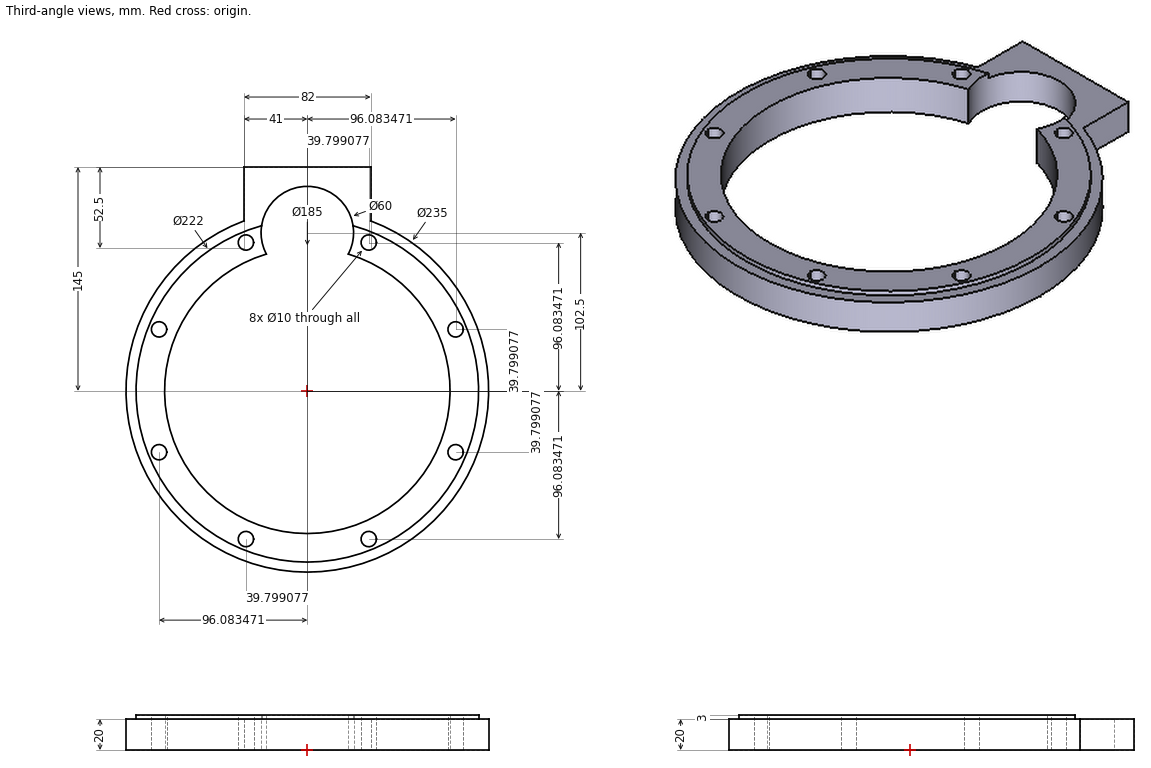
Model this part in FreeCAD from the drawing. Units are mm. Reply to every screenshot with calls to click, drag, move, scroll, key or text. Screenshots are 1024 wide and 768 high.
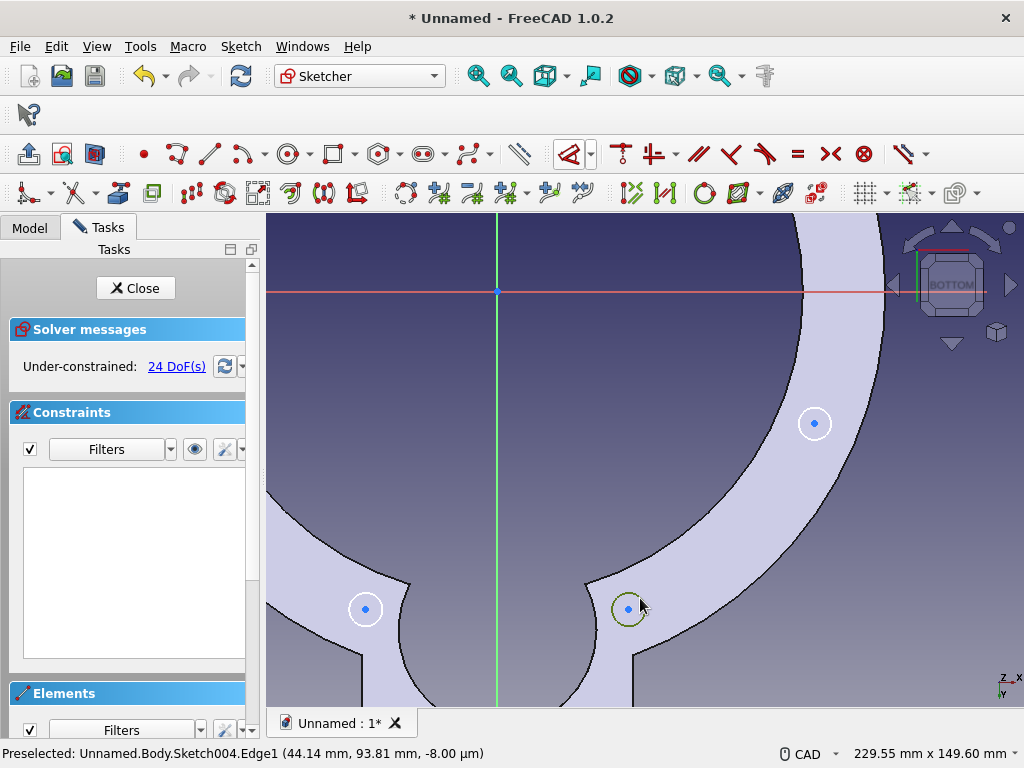
click(826, 412)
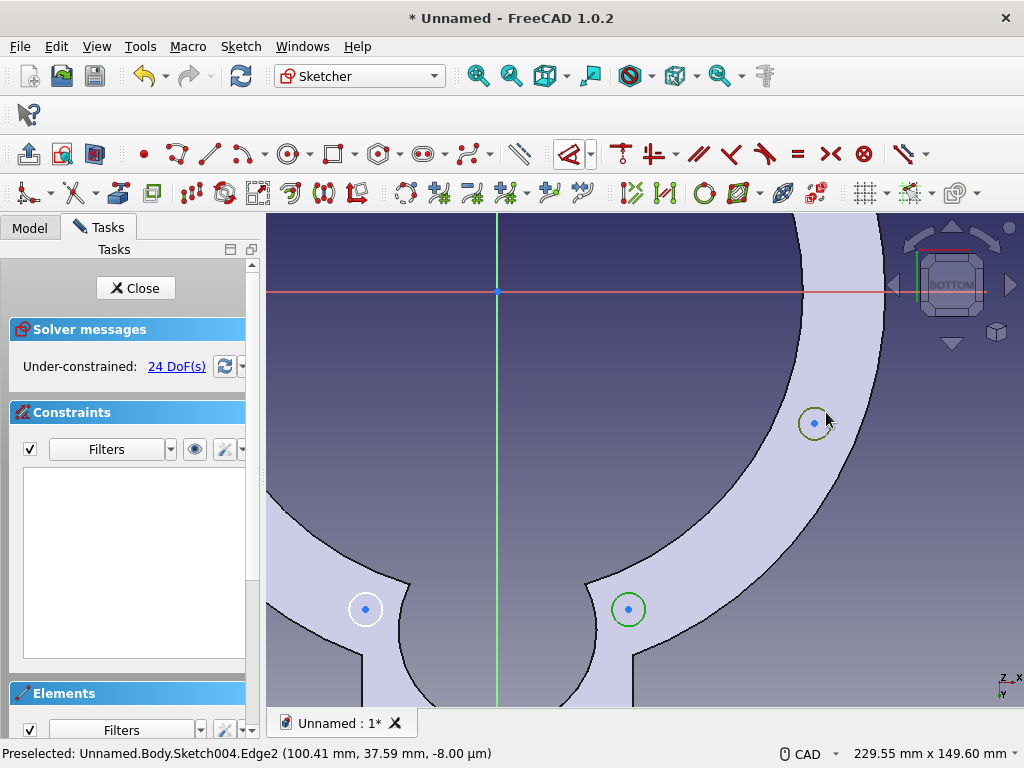
scroll(641, 597, down, 4)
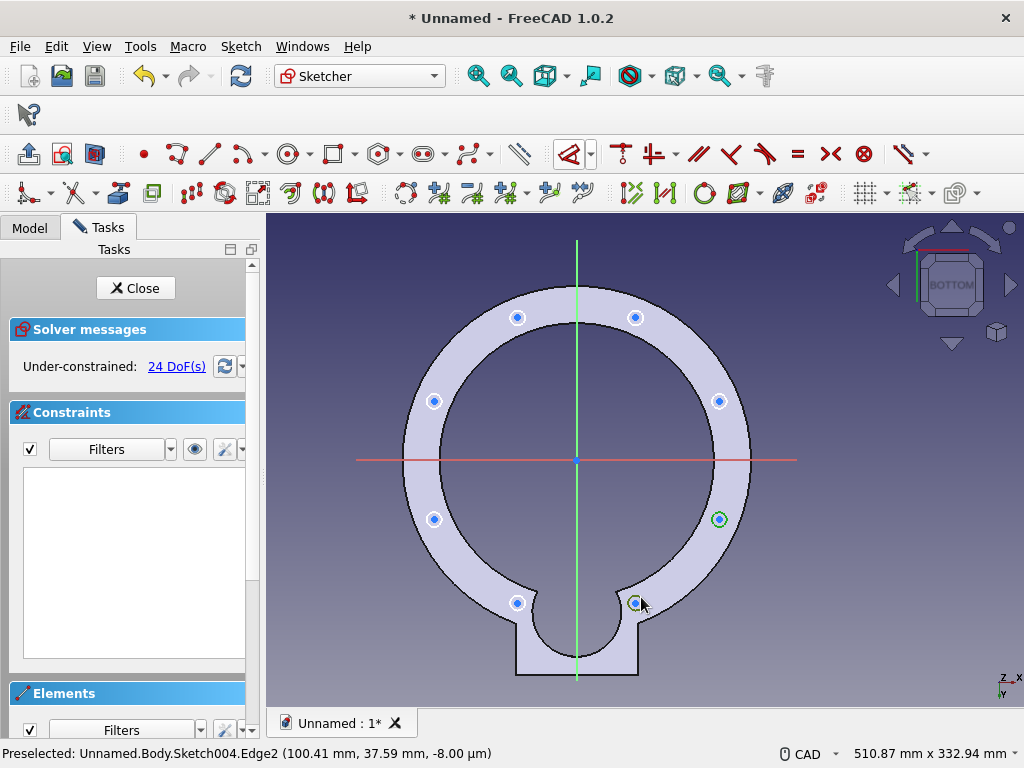
scroll(725, 396, up, 4)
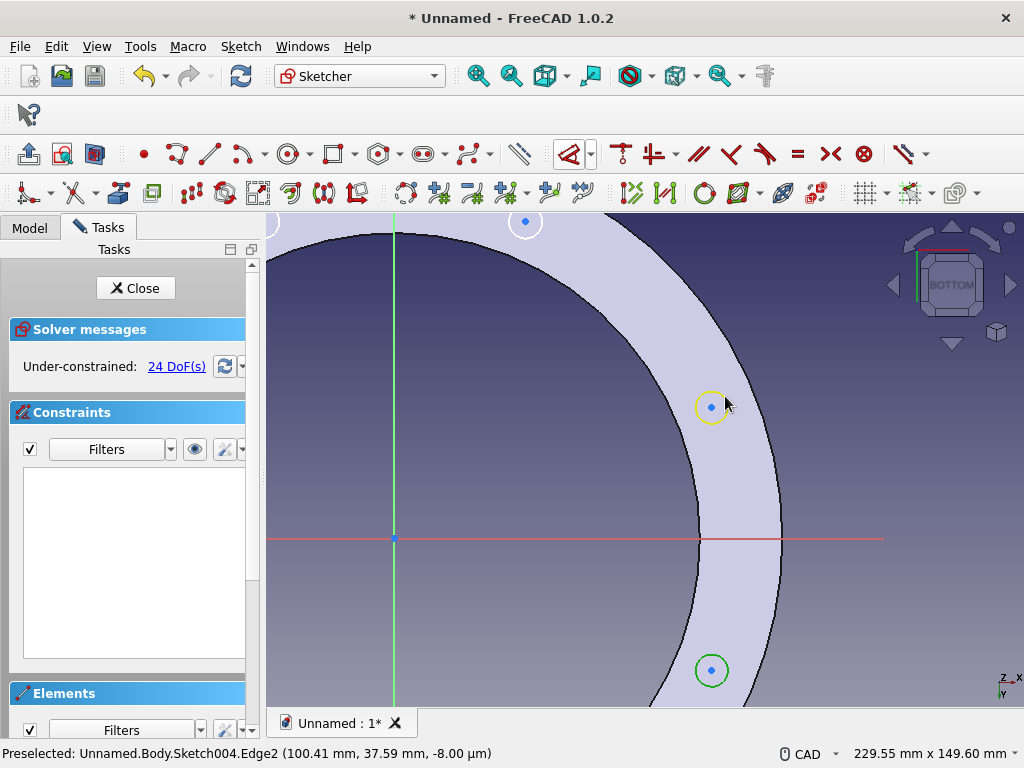
click(723, 396)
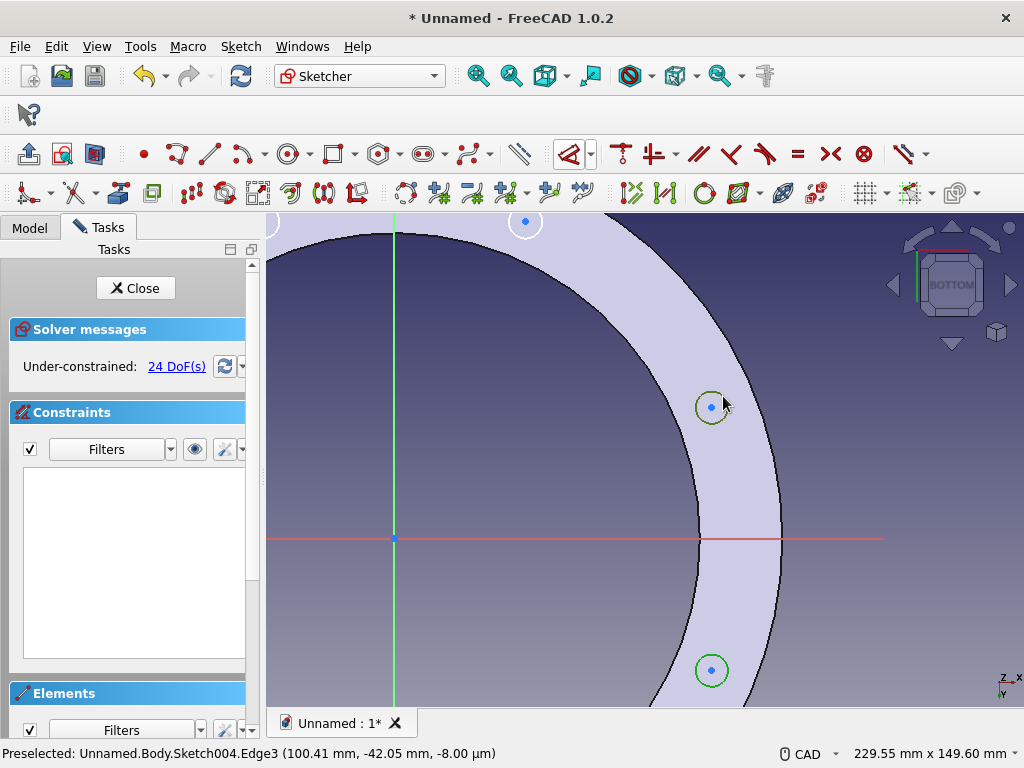
scroll(725, 396, down, 4)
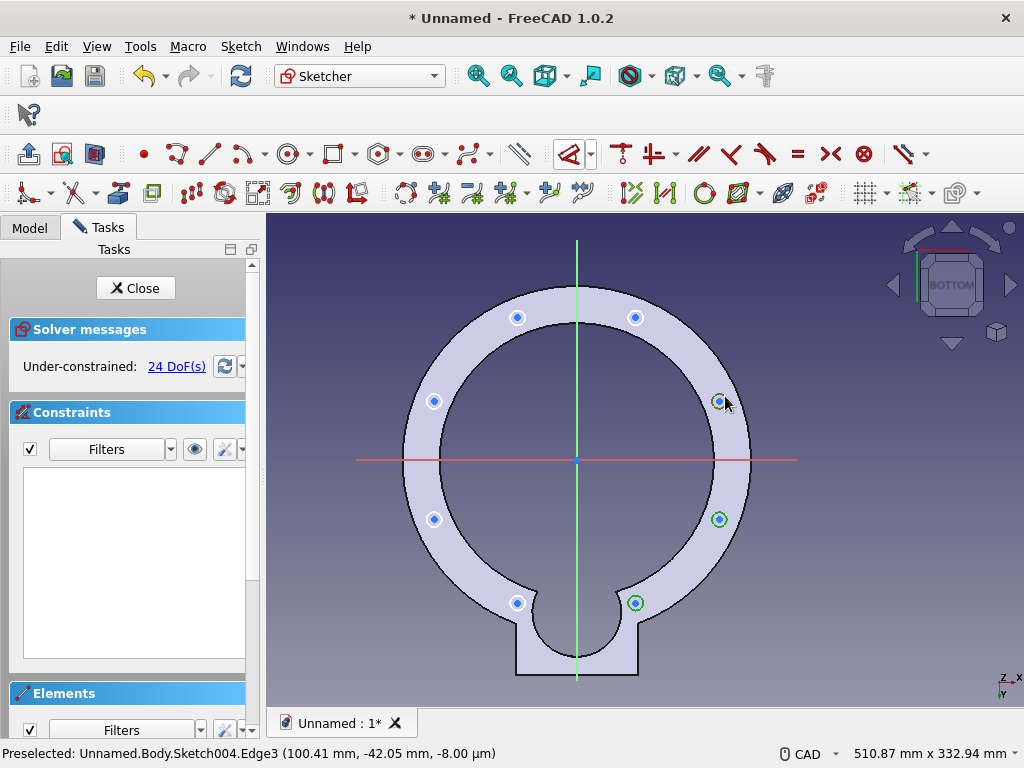
scroll(641, 313, up, 4)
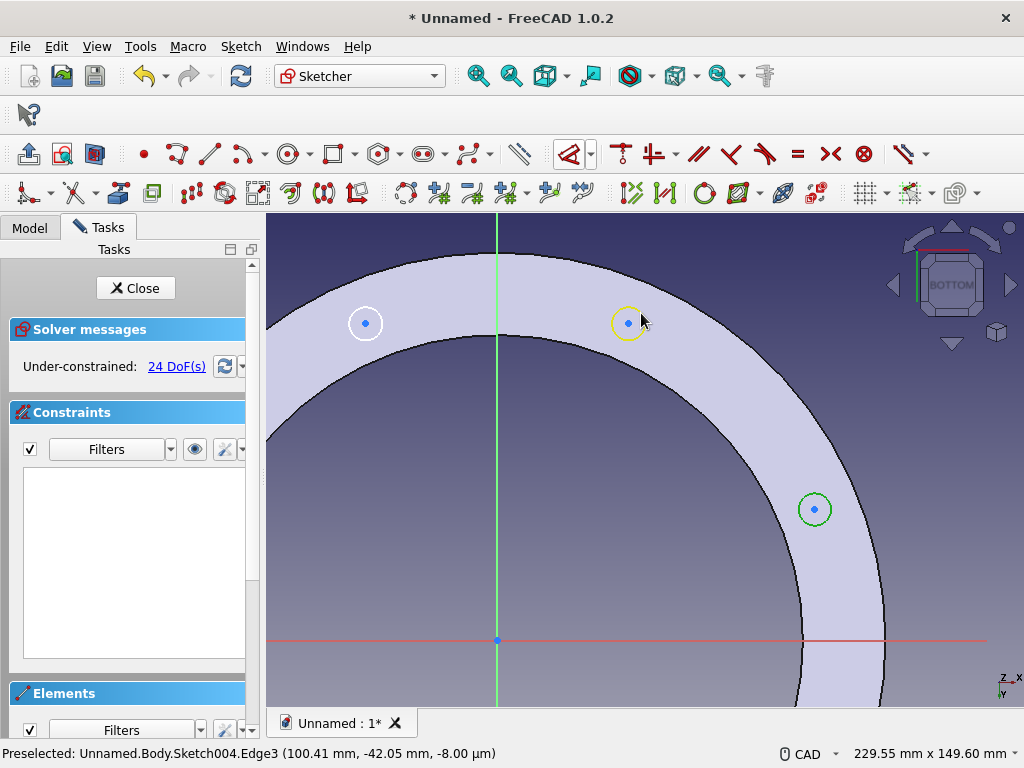
click(640, 312)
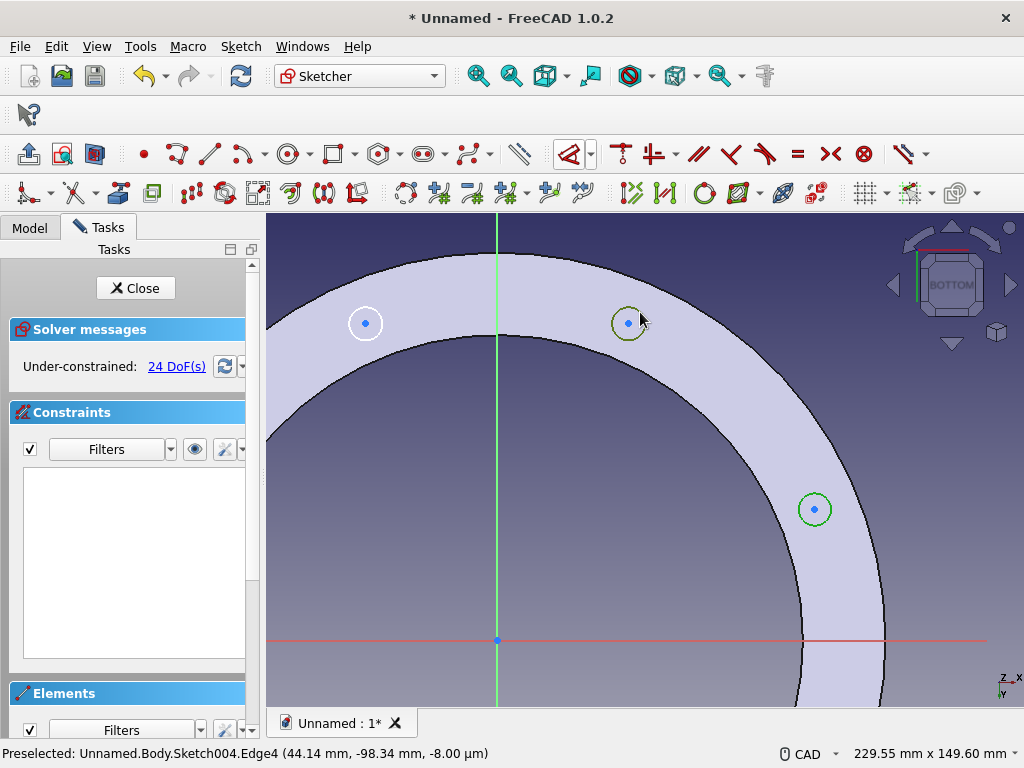
click(378, 312)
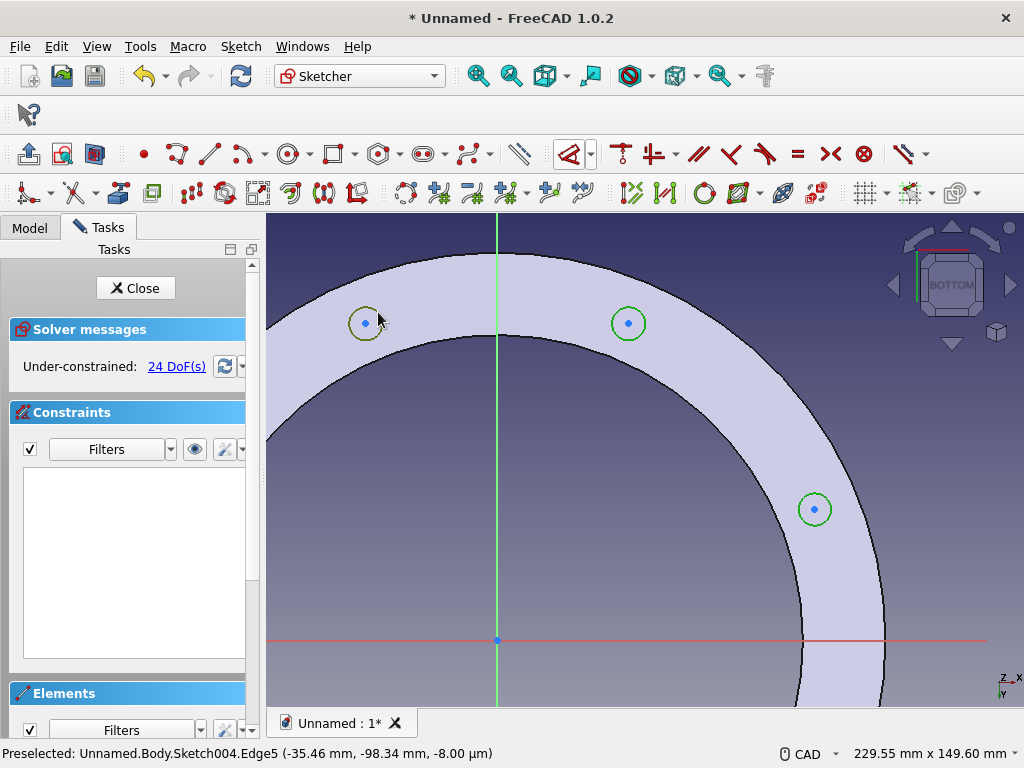
scroll(641, 313, down, 4)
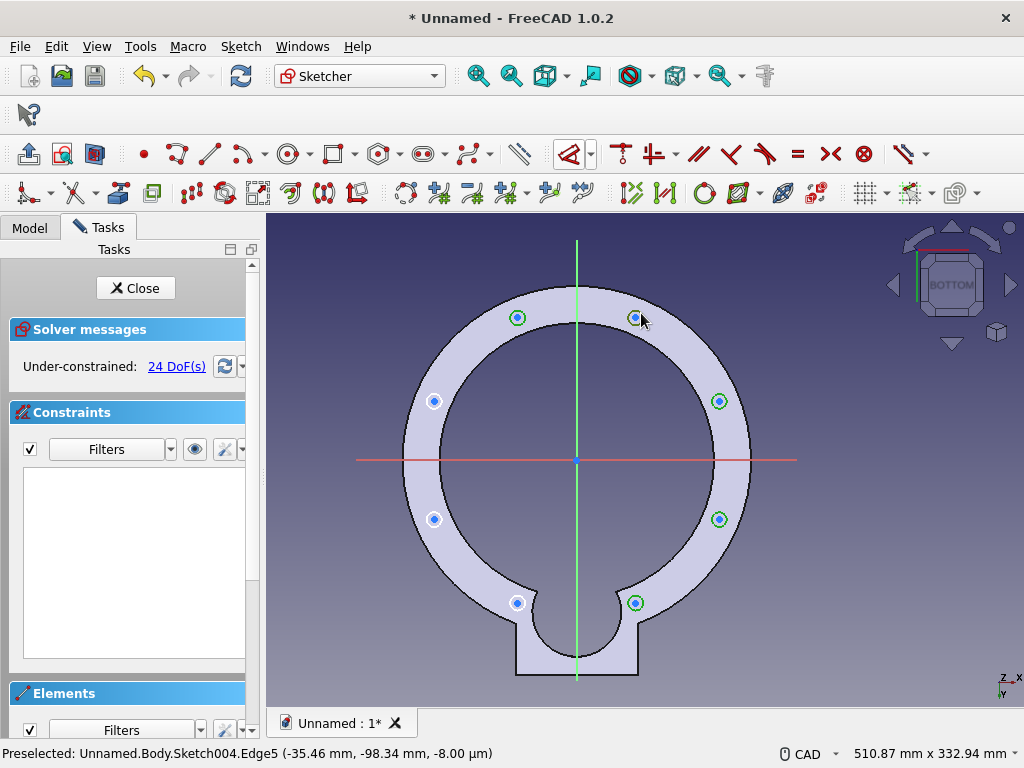
scroll(439, 396, up, 4)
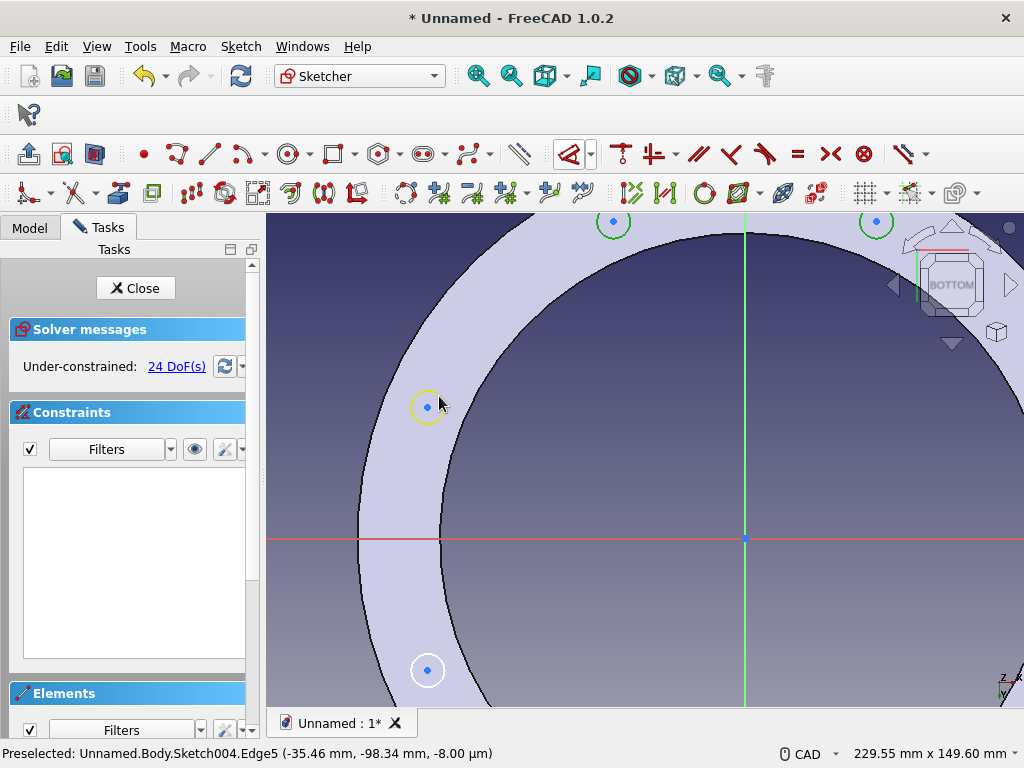
click(440, 396)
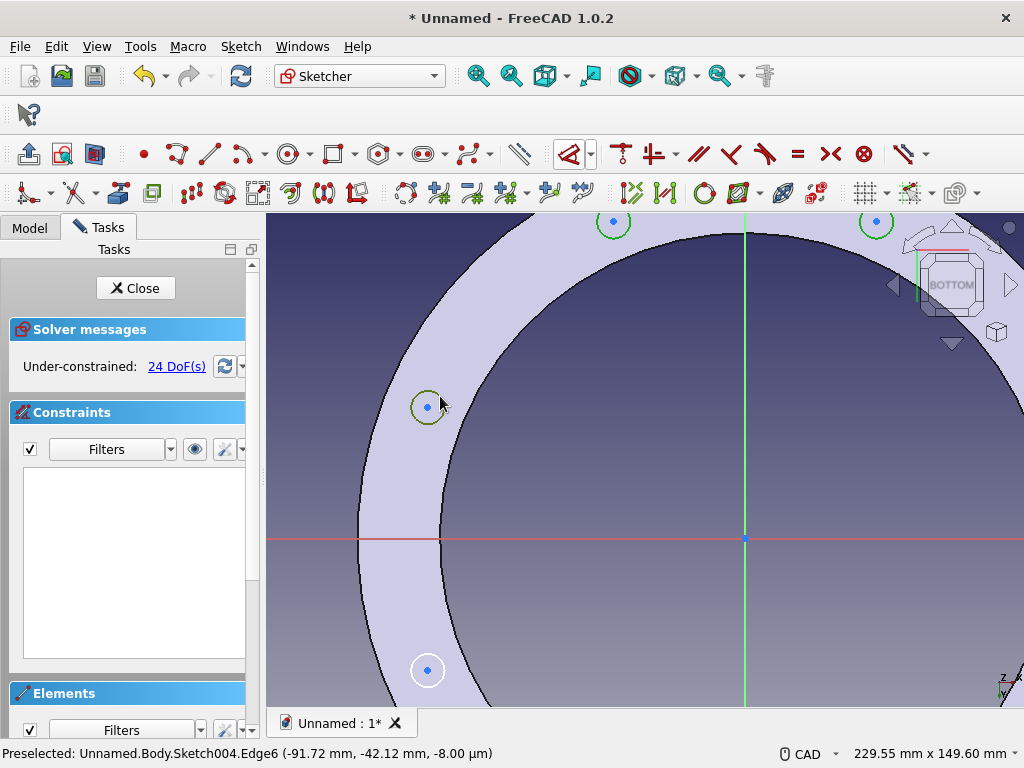
click(440, 659)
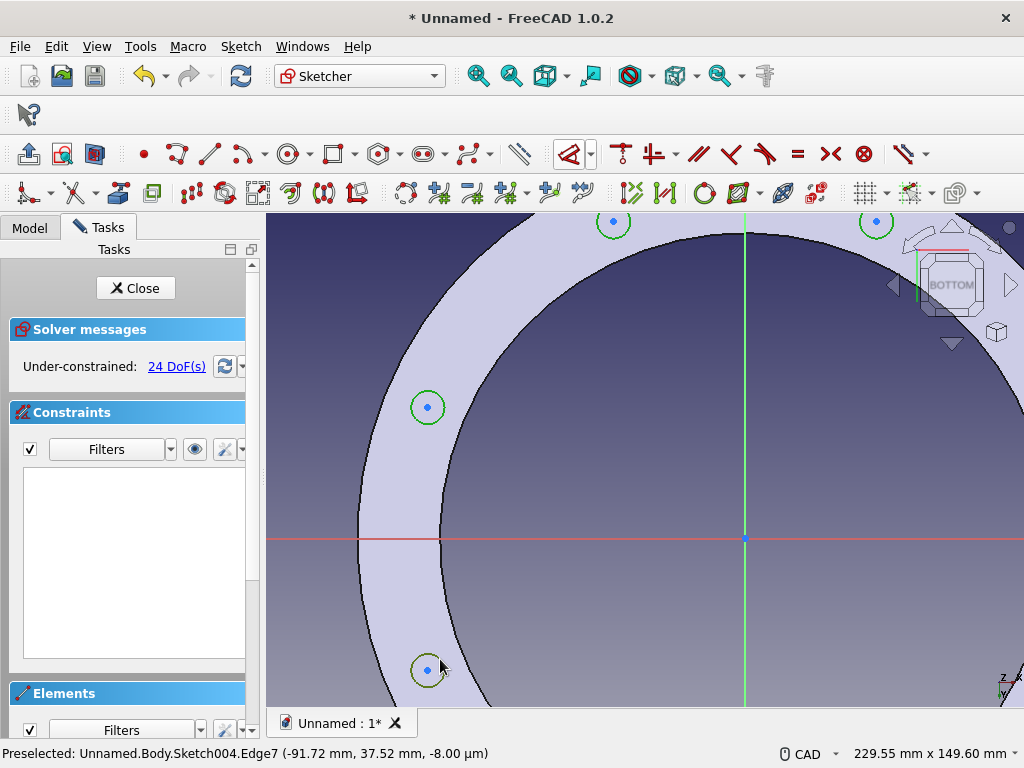
scroll(439, 396, down, 4)